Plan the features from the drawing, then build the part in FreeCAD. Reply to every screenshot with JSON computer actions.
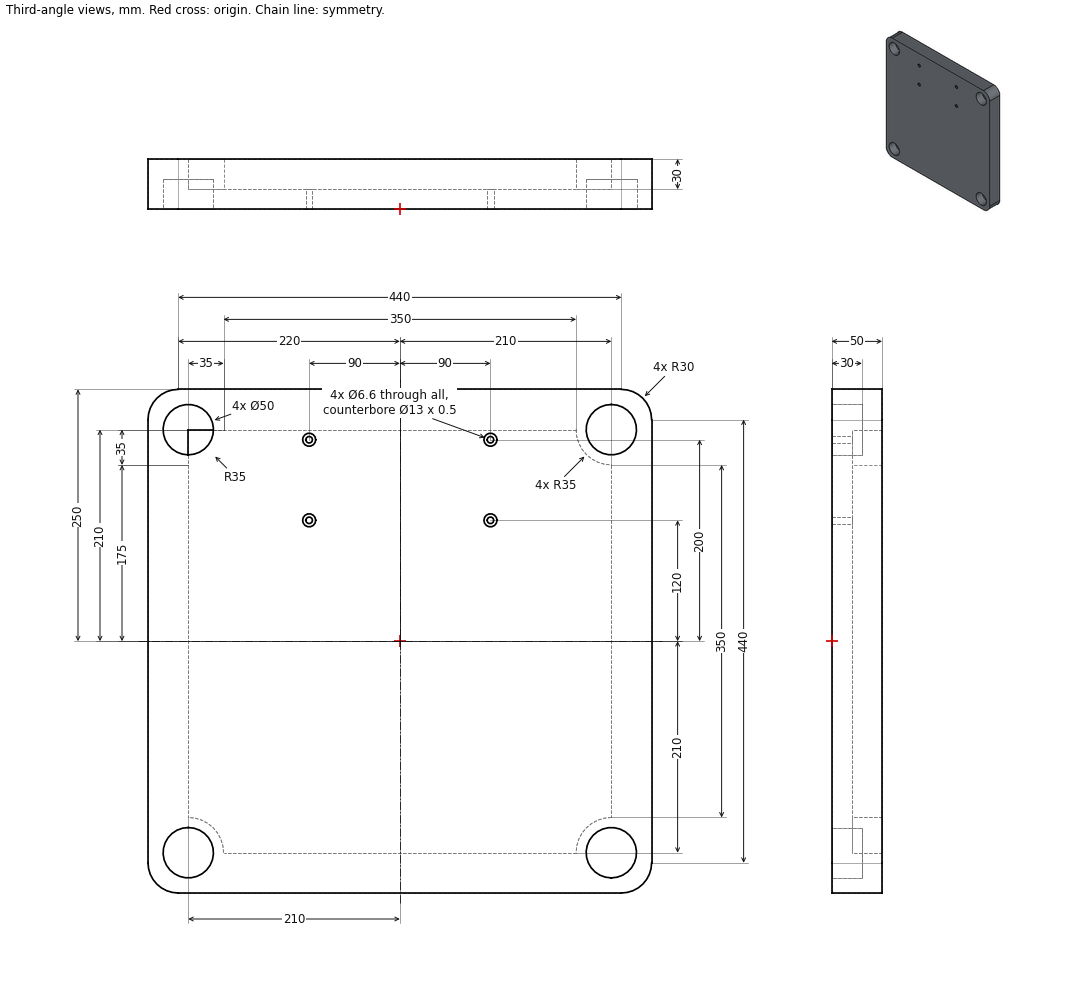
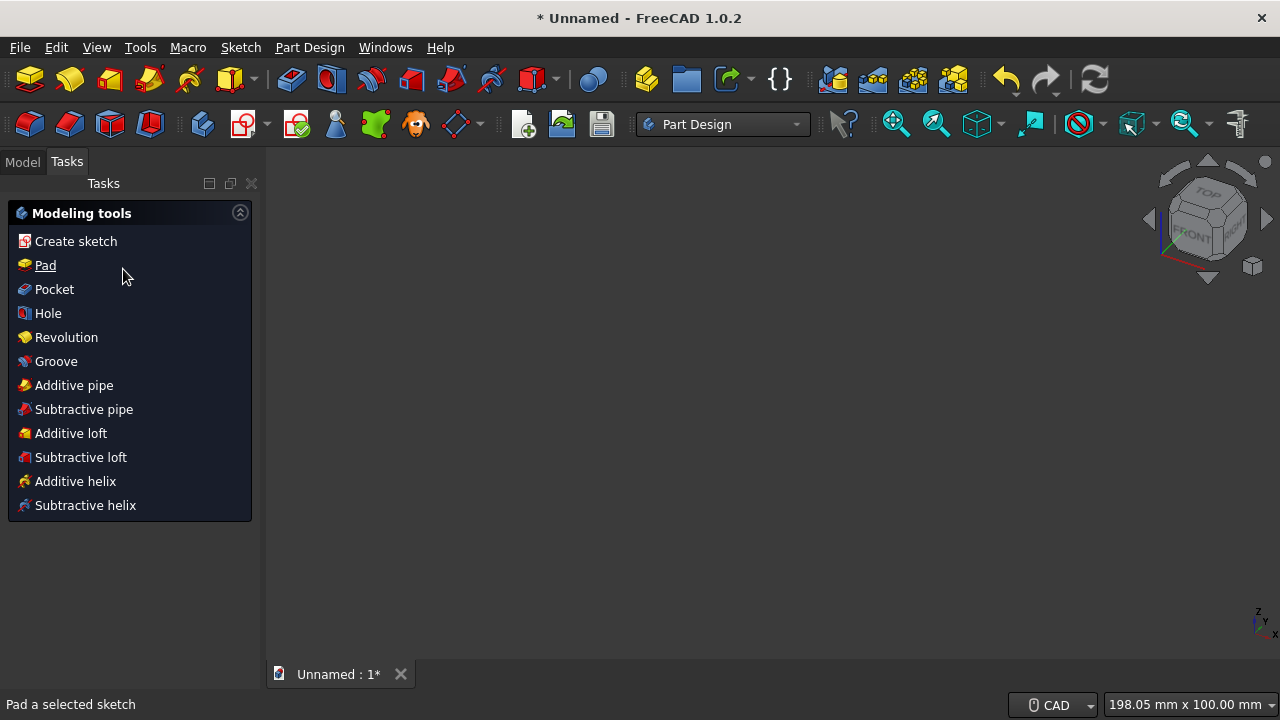
{"action": "left_click", "coordinate": [30, 80]}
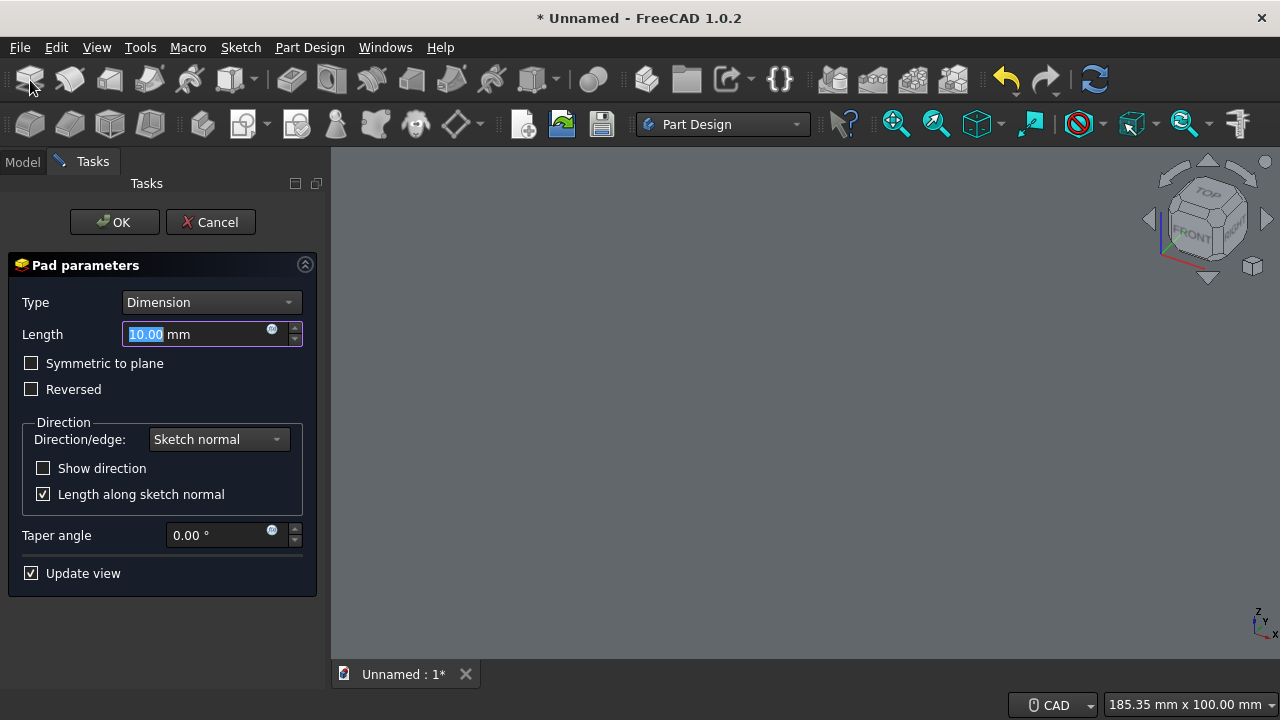
{"action": "type", "text": "50"}
{"action": "key", "text": "Tab"}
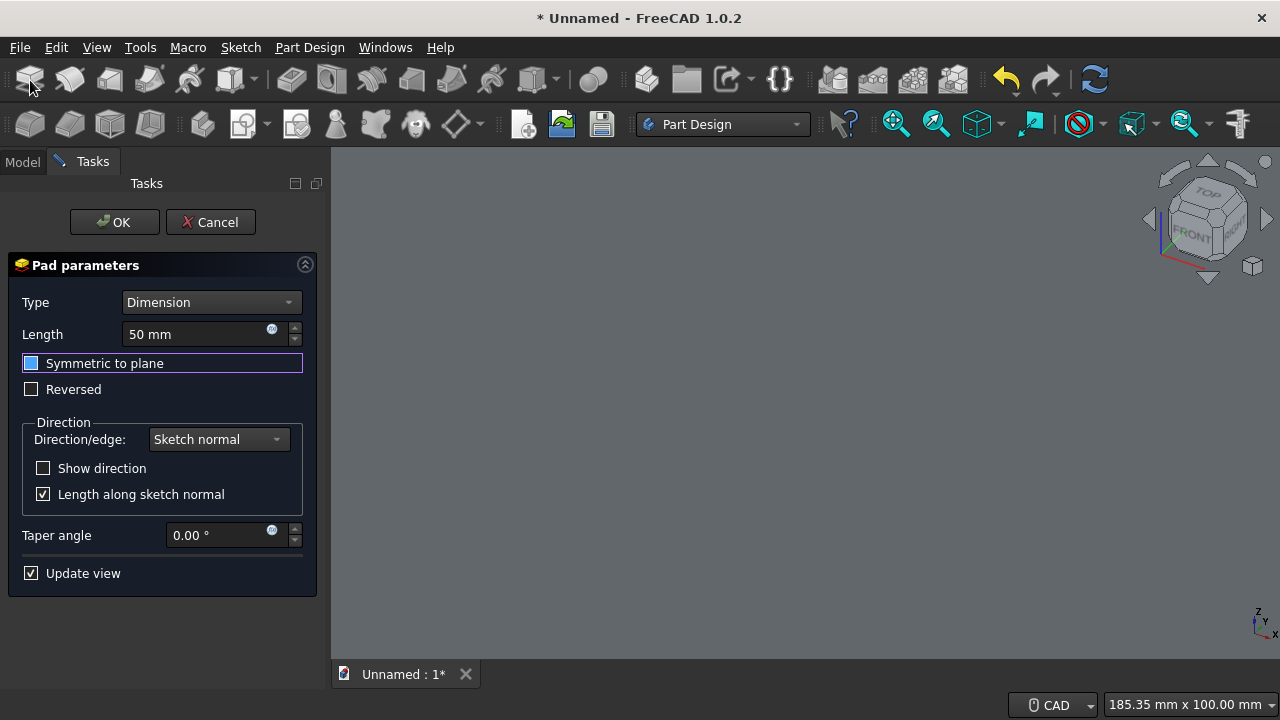
{"action": "left_click", "coordinate": [30, 389]}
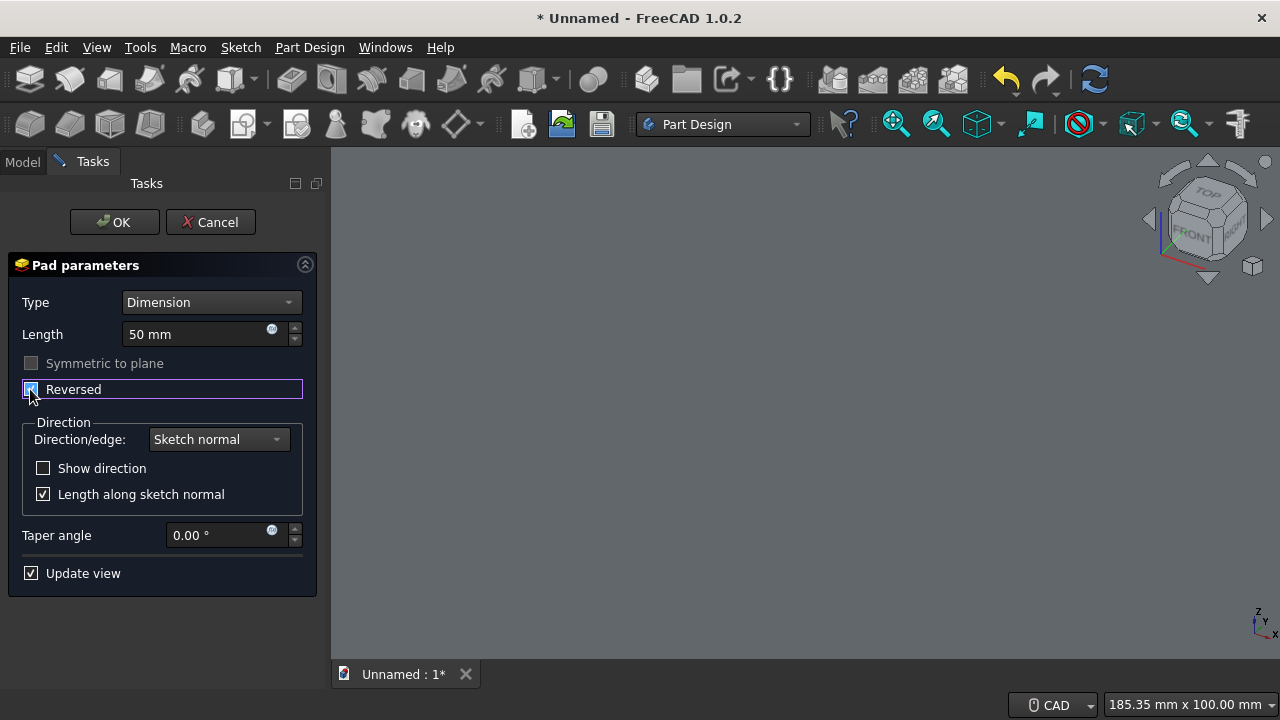
{"action": "left_click", "coordinate": [115, 222]}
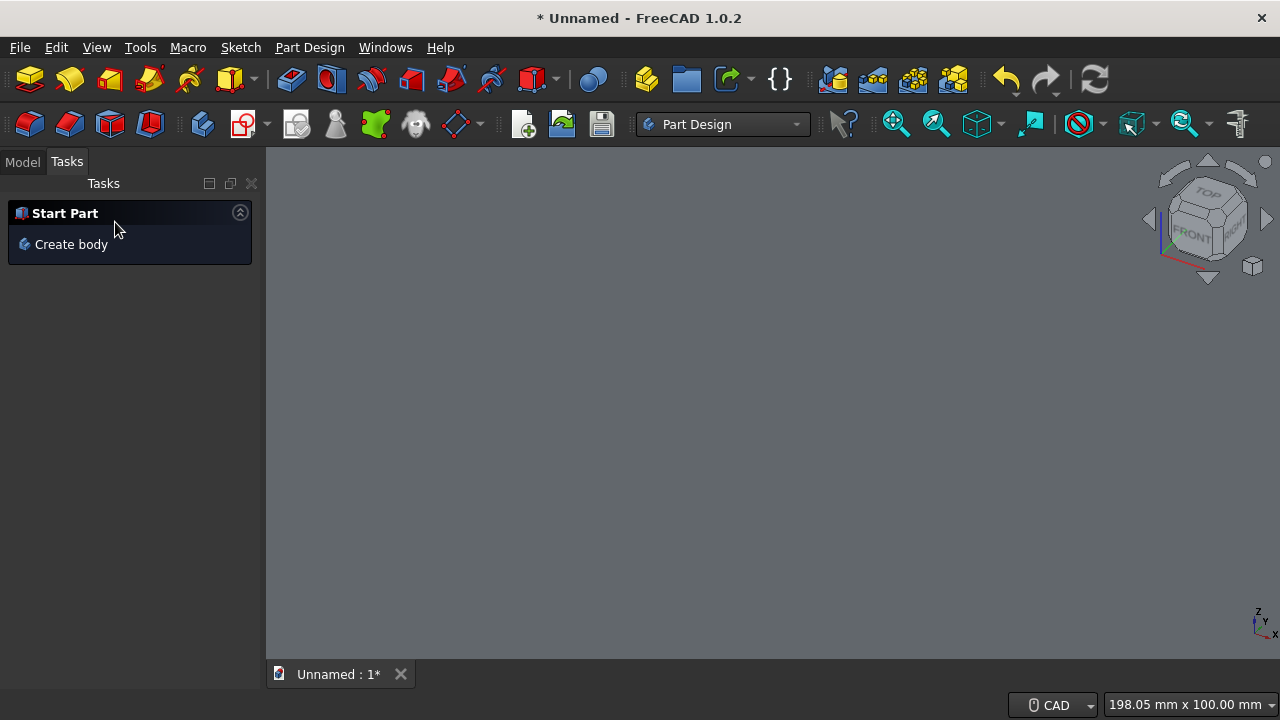
{"action": "key", "text": "v f"}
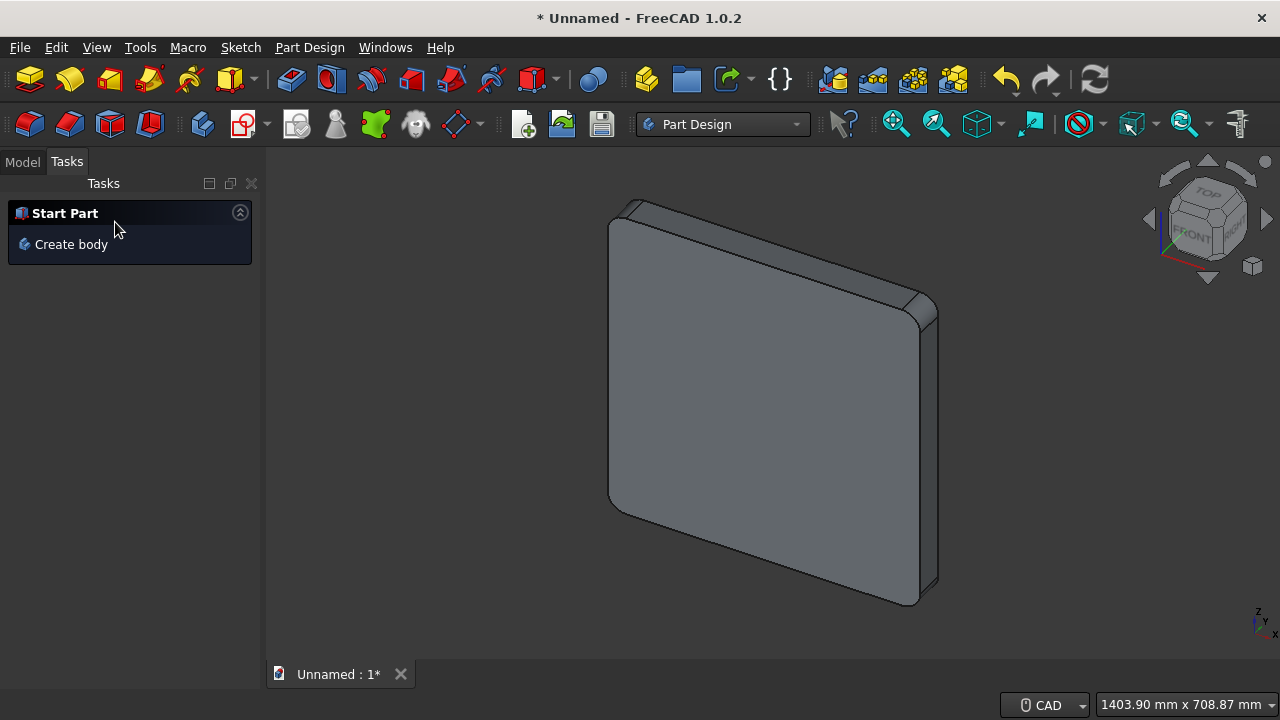
{"action": "key", "text": "4"}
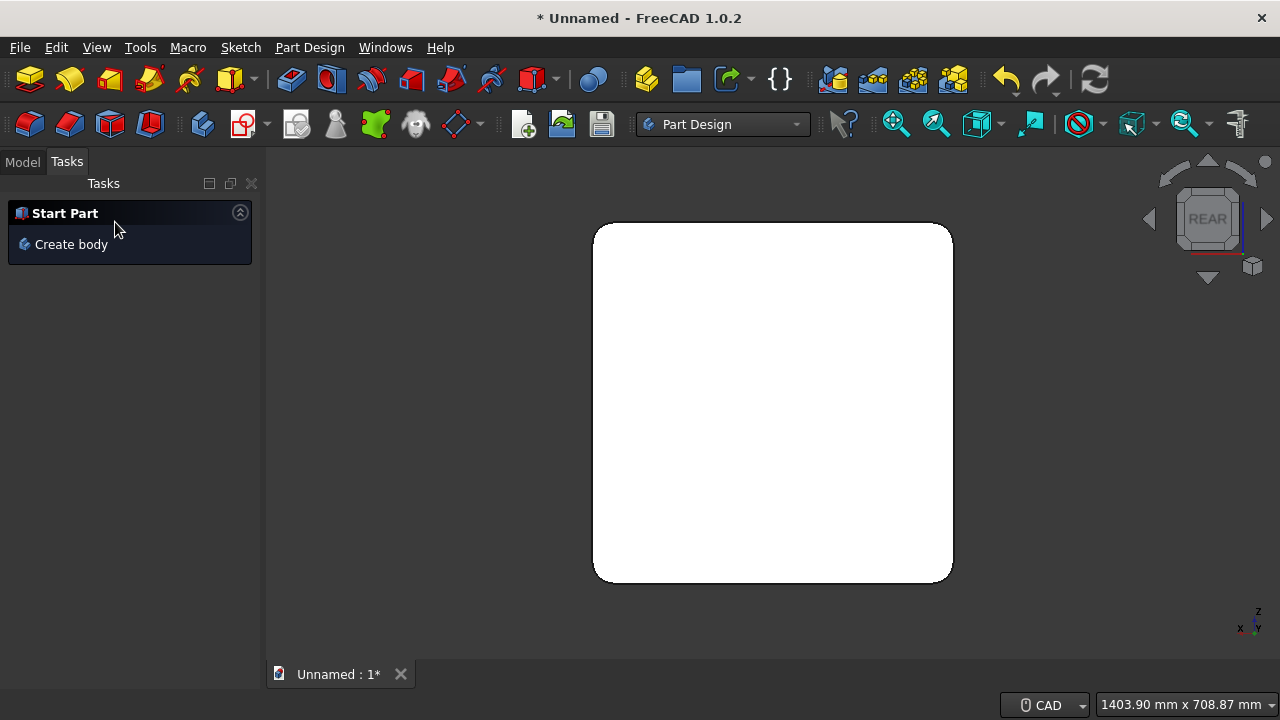
{"action": "left_click", "coordinate": [773, 402]}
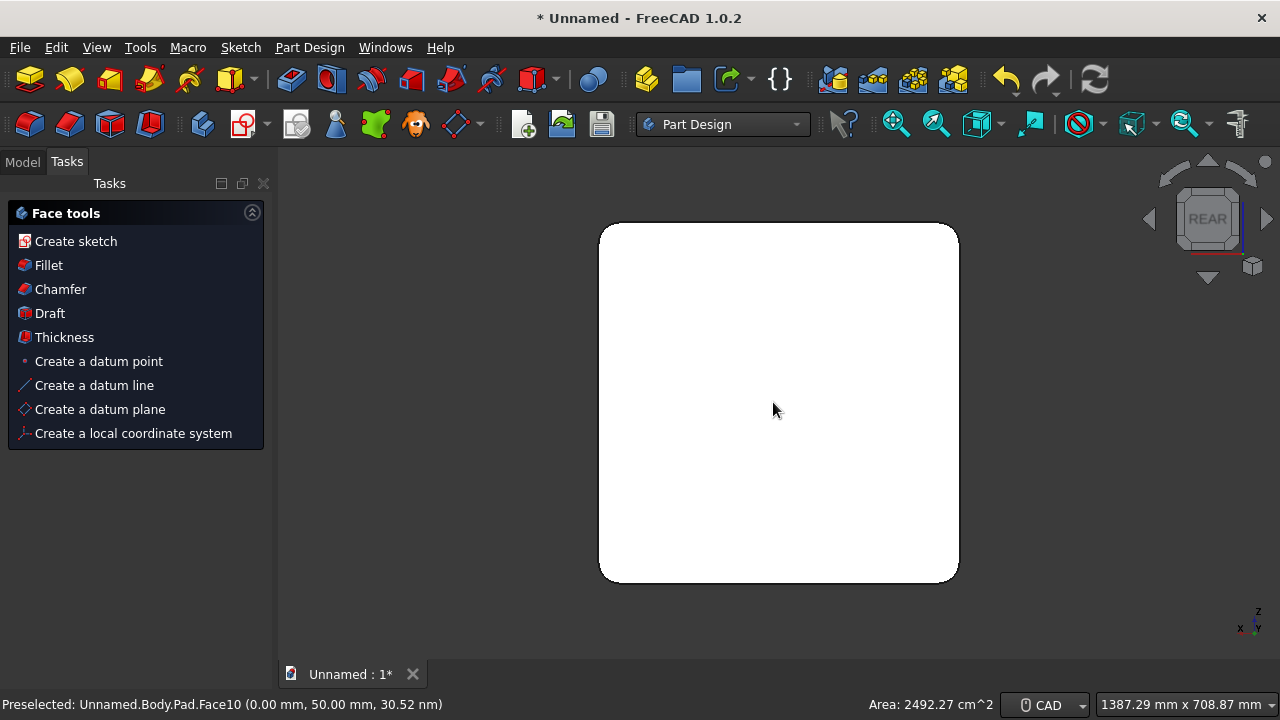
{"action": "left_click", "coordinate": [244, 124]}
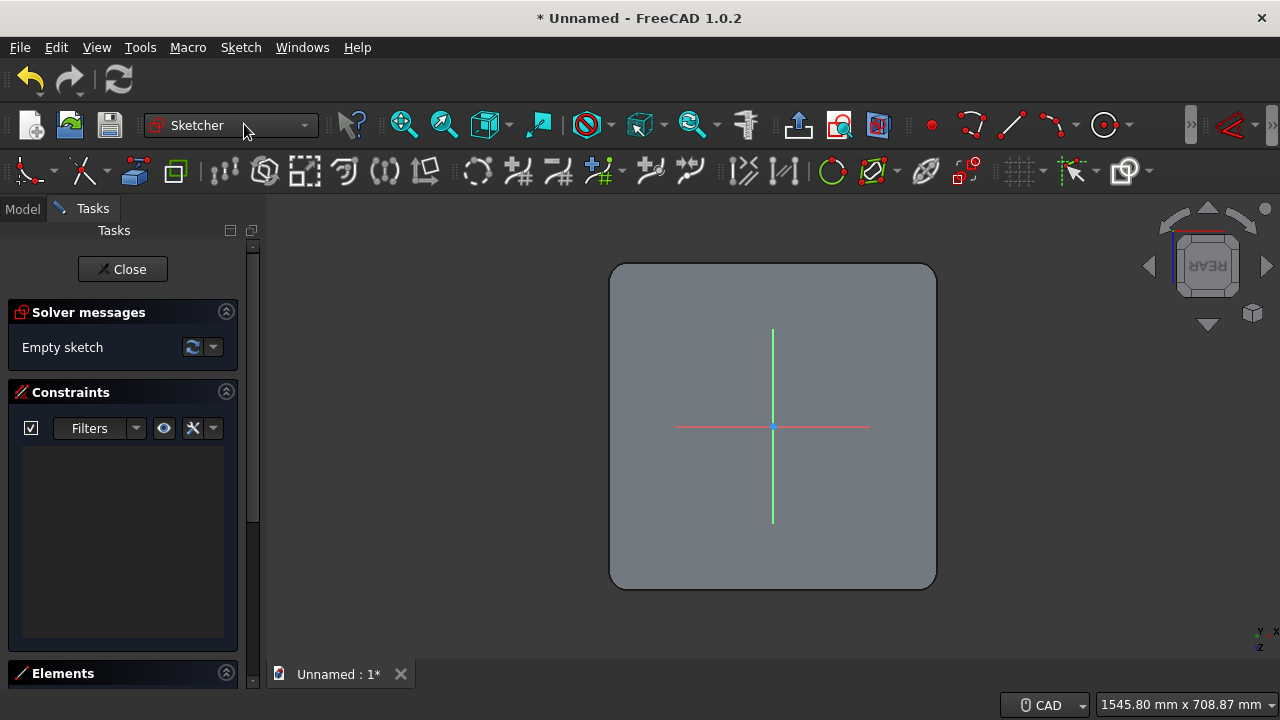
{"action": "key", "text": "g l"}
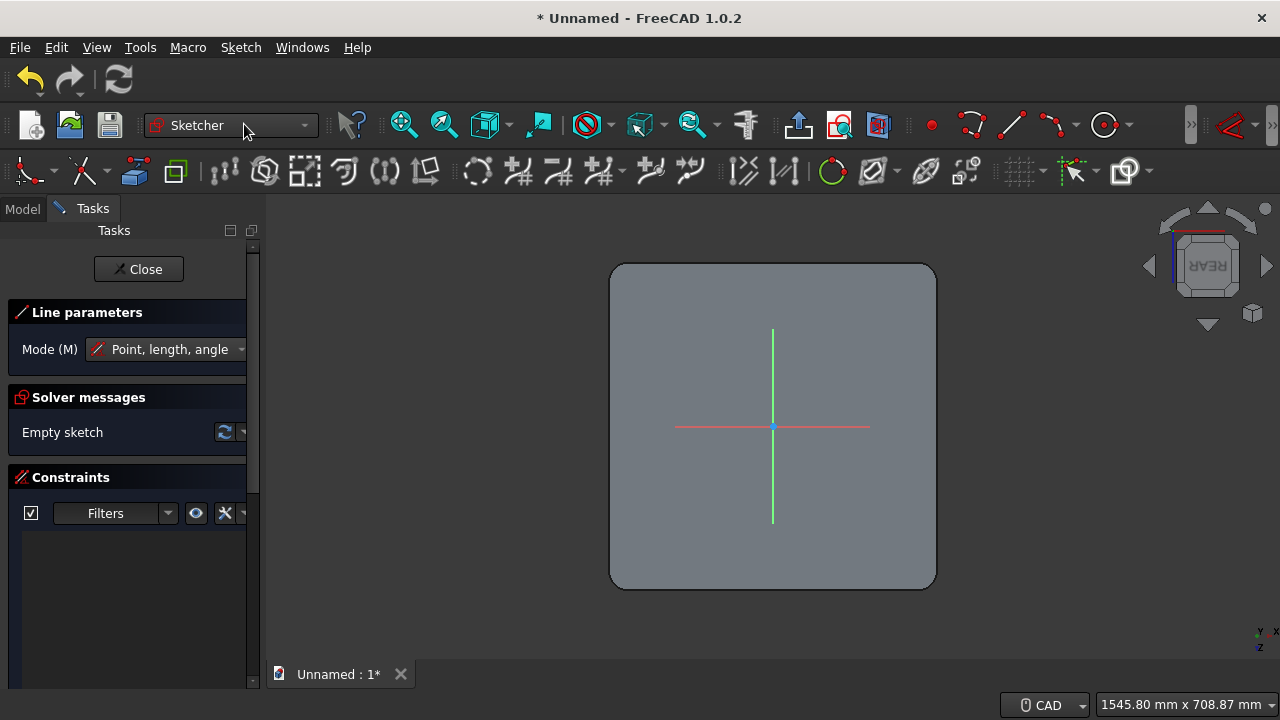
{"action": "left_click", "coordinate": [658, 564]}
{"action": "left_click", "coordinate": [888, 564]}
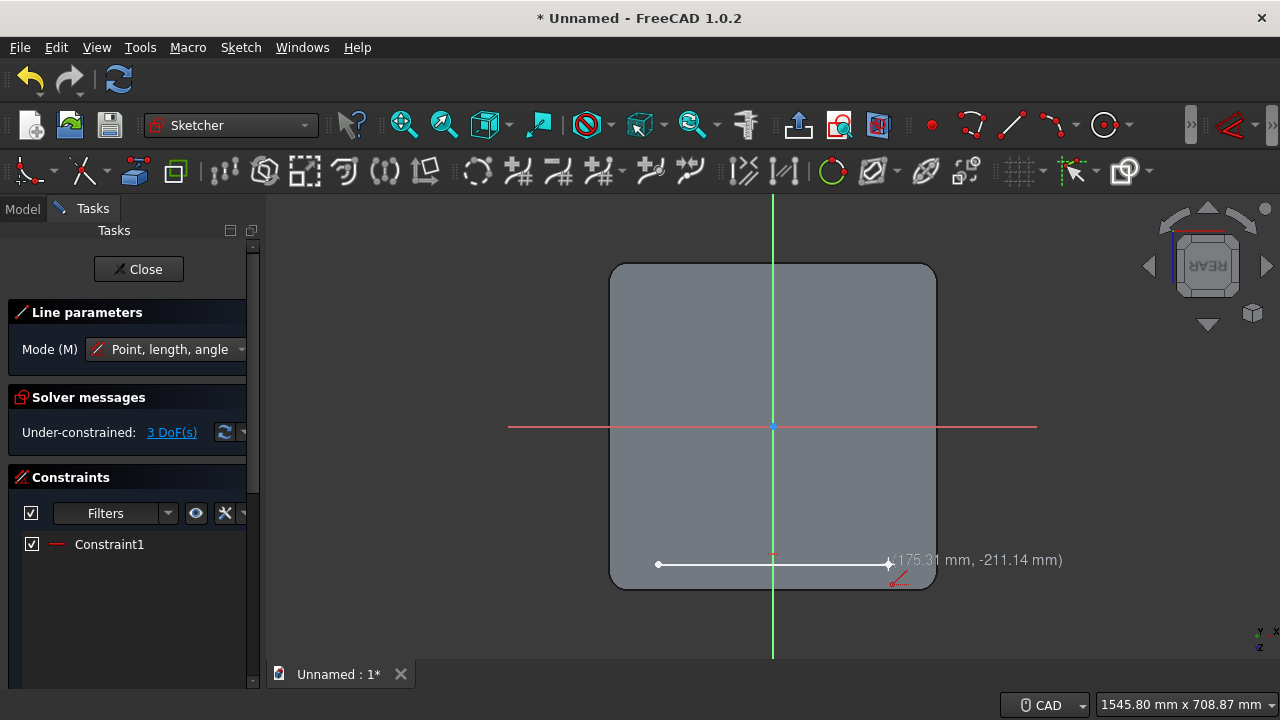
{"action": "left_click", "coordinate": [911, 541]}
{"action": "left_click", "coordinate": [911, 312]}